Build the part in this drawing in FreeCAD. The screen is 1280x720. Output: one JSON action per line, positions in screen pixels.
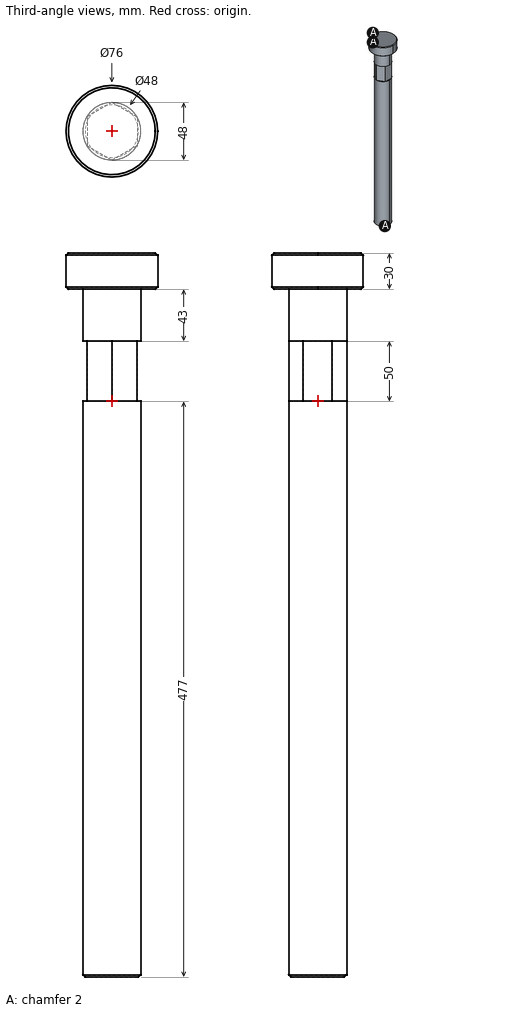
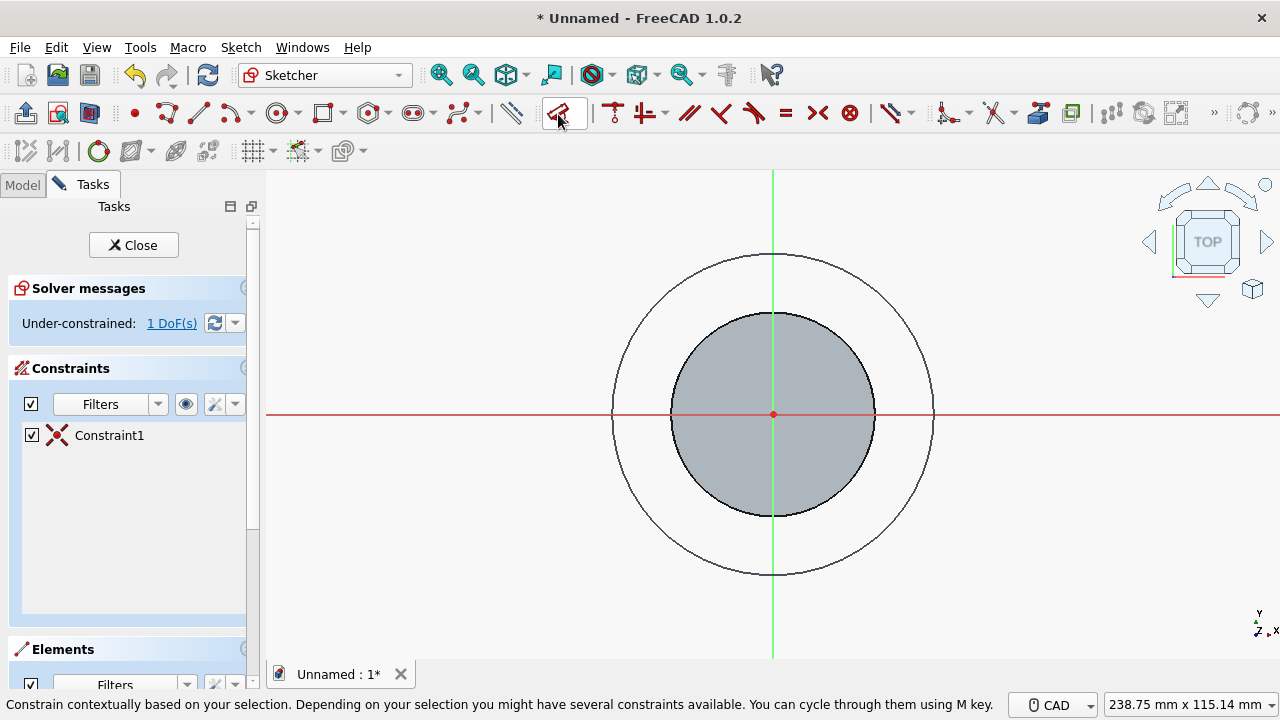
{"action": "left_click", "coordinate": [886, 300]}
{"action": "left_click", "coordinate": [908, 277]}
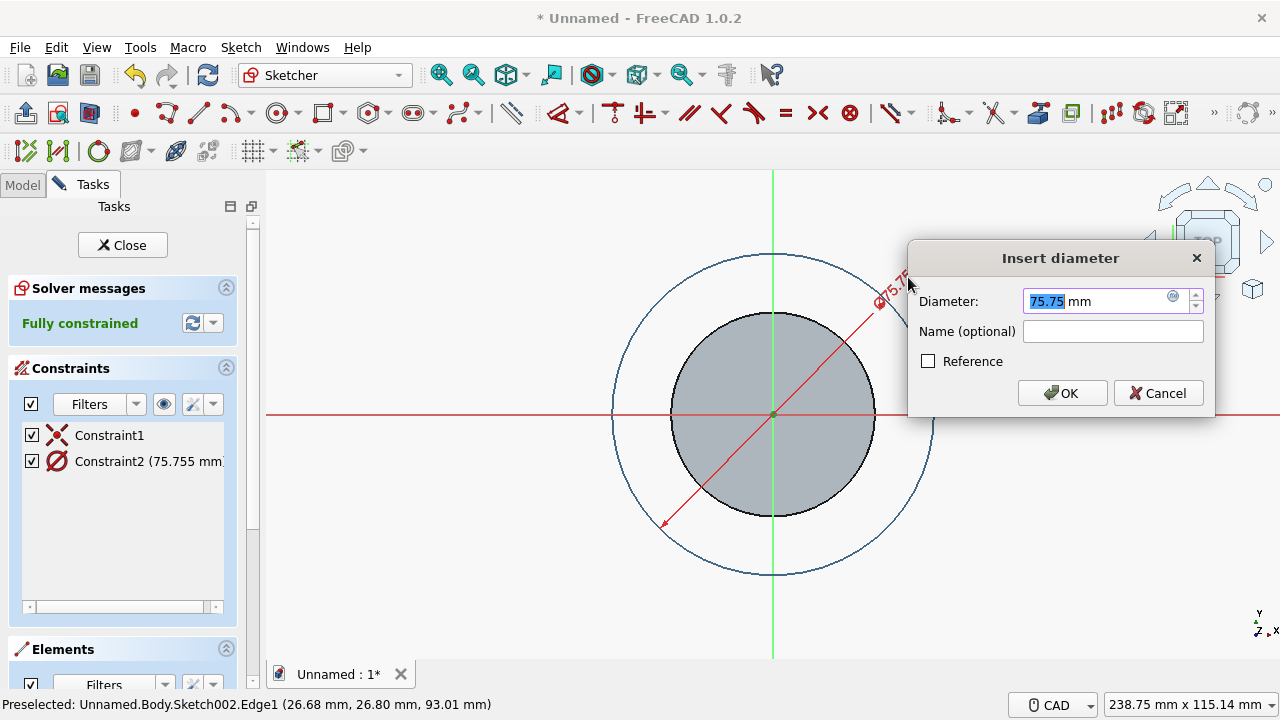
{"action": "type", "text": "76"}
{"action": "key", "text": "Return"}
{"action": "key", "text": "Escape"}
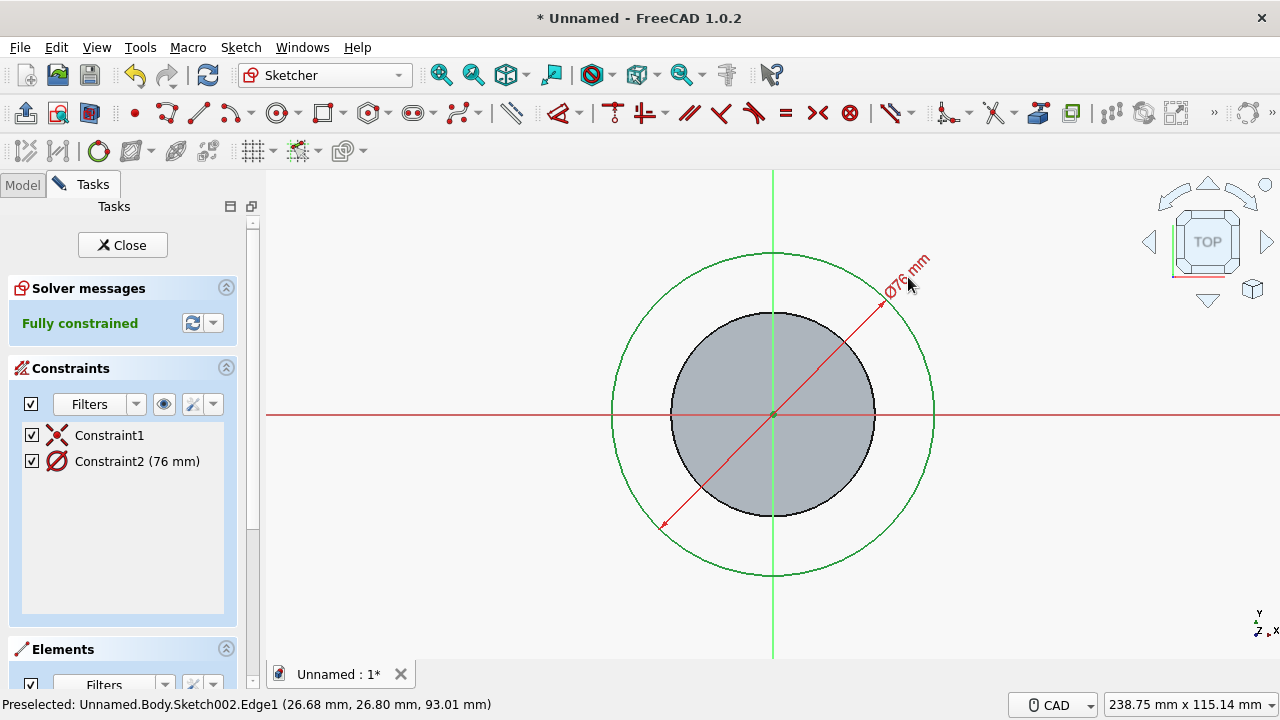
{"action": "left_click", "coordinate": [123, 245]}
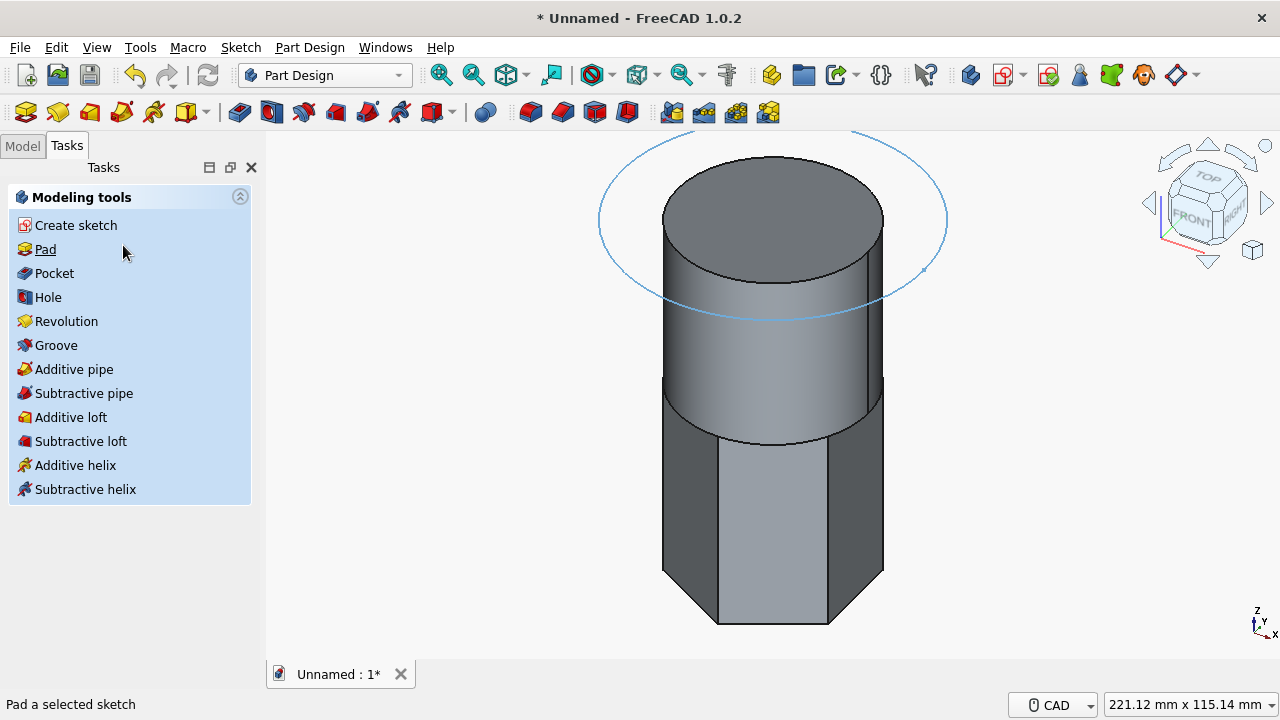
{"action": "left_click", "coordinate": [26, 112]}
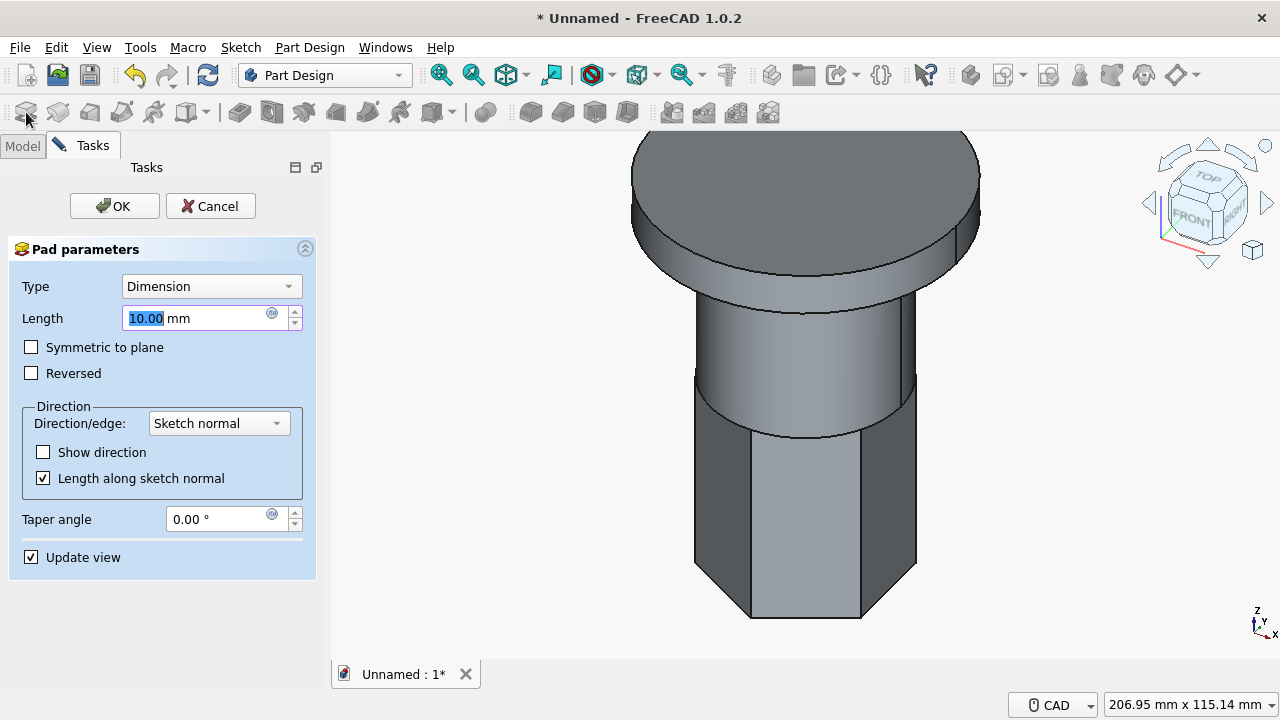
{"action": "type", "text": "30"}
{"action": "key", "text": "Tab"}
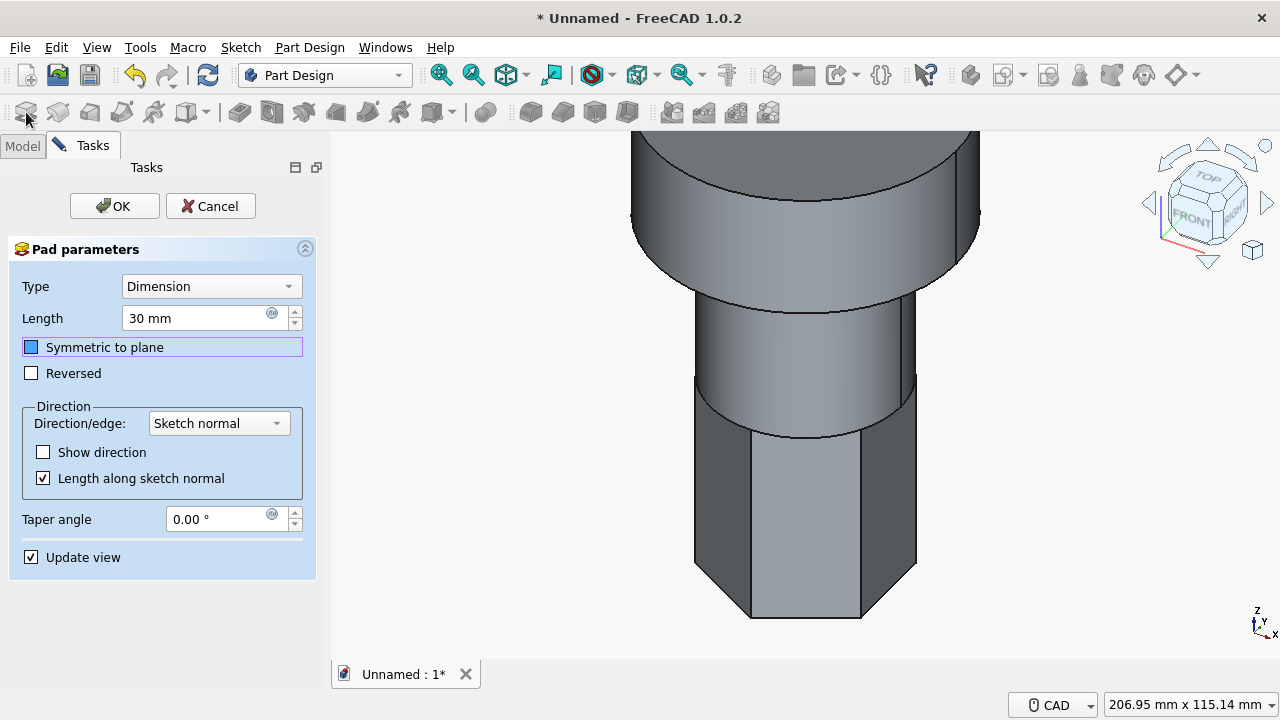
{"action": "left_click", "coordinate": [115, 206]}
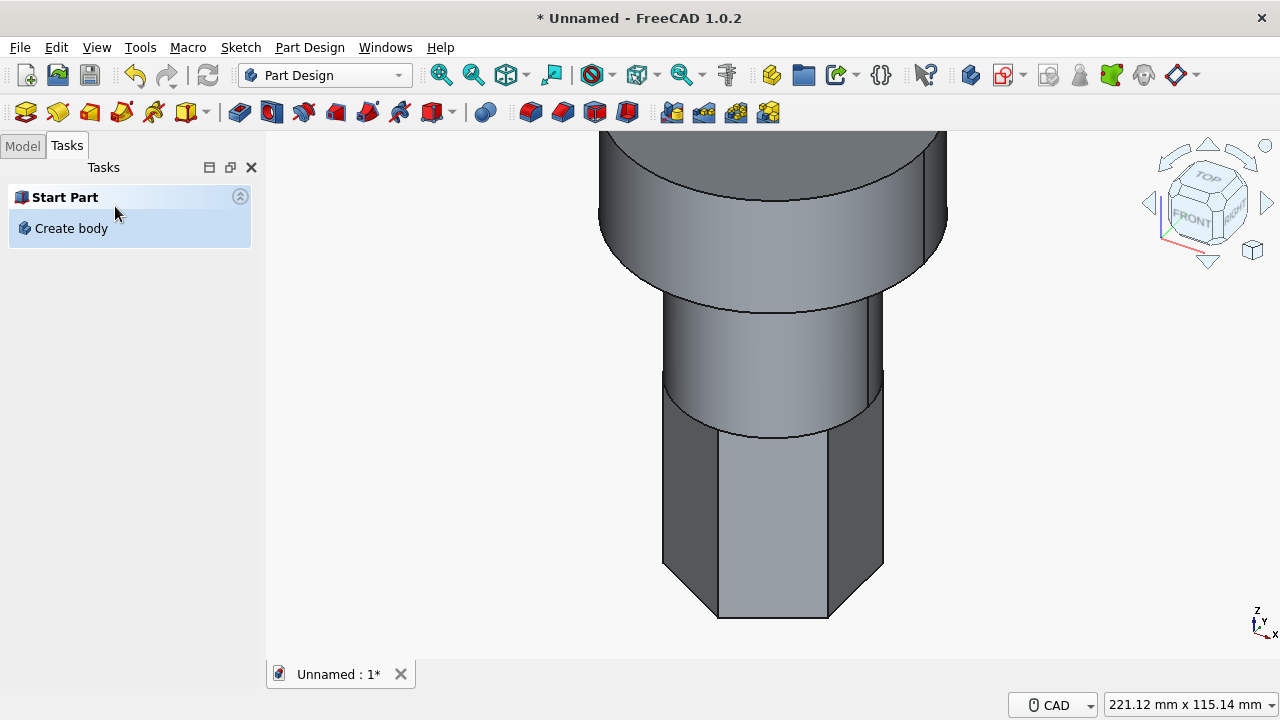
{"action": "key", "text": "v f"}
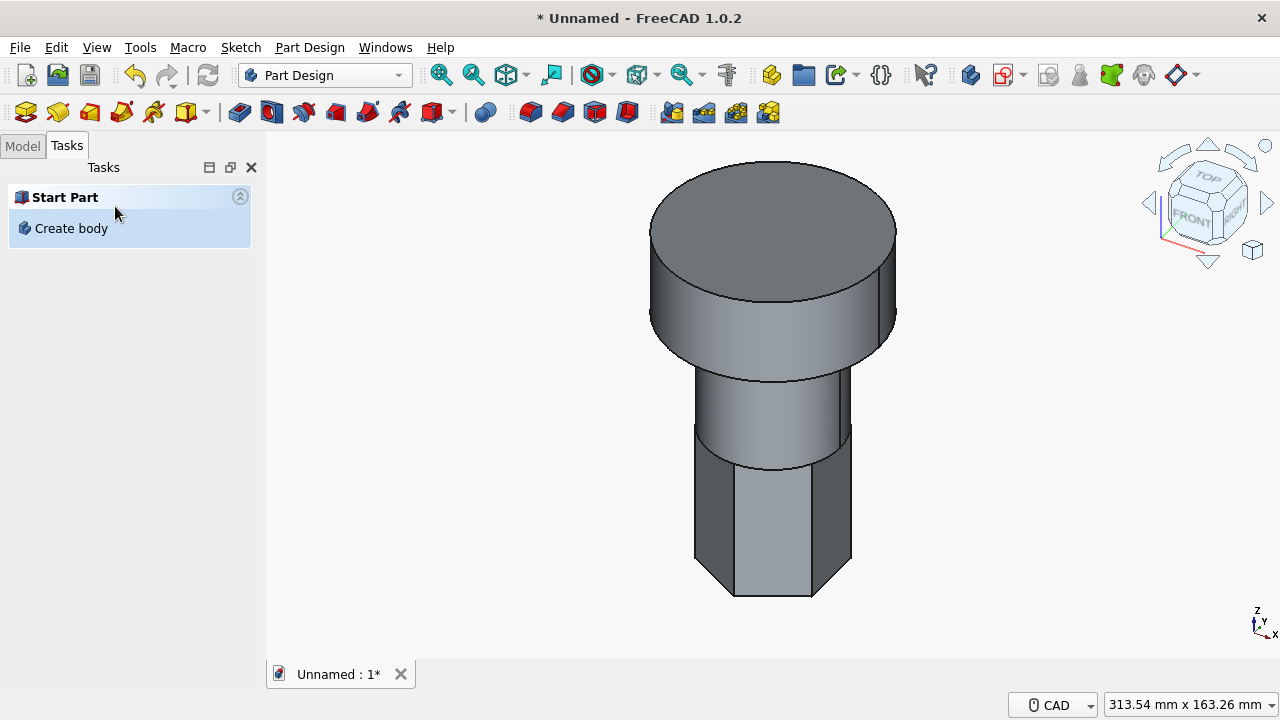
{"action": "left_click", "coordinate": [23, 145]}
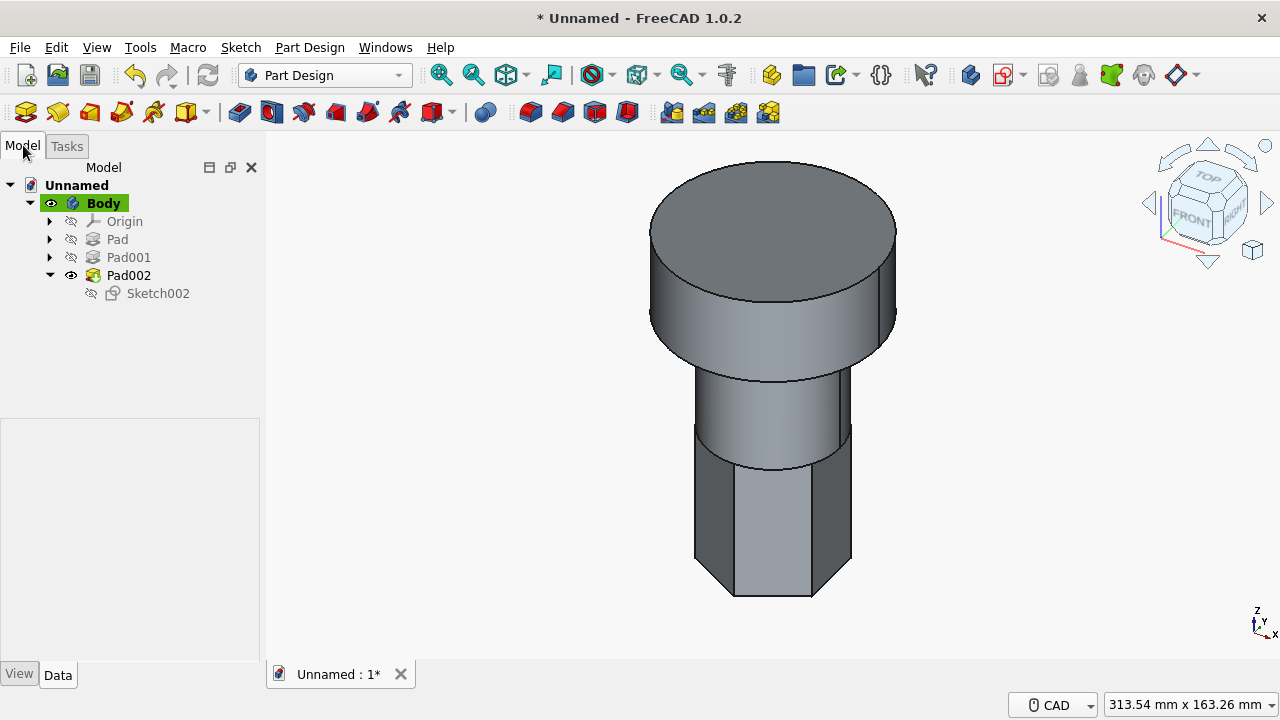
{"action": "left_click", "coordinate": [50, 221]}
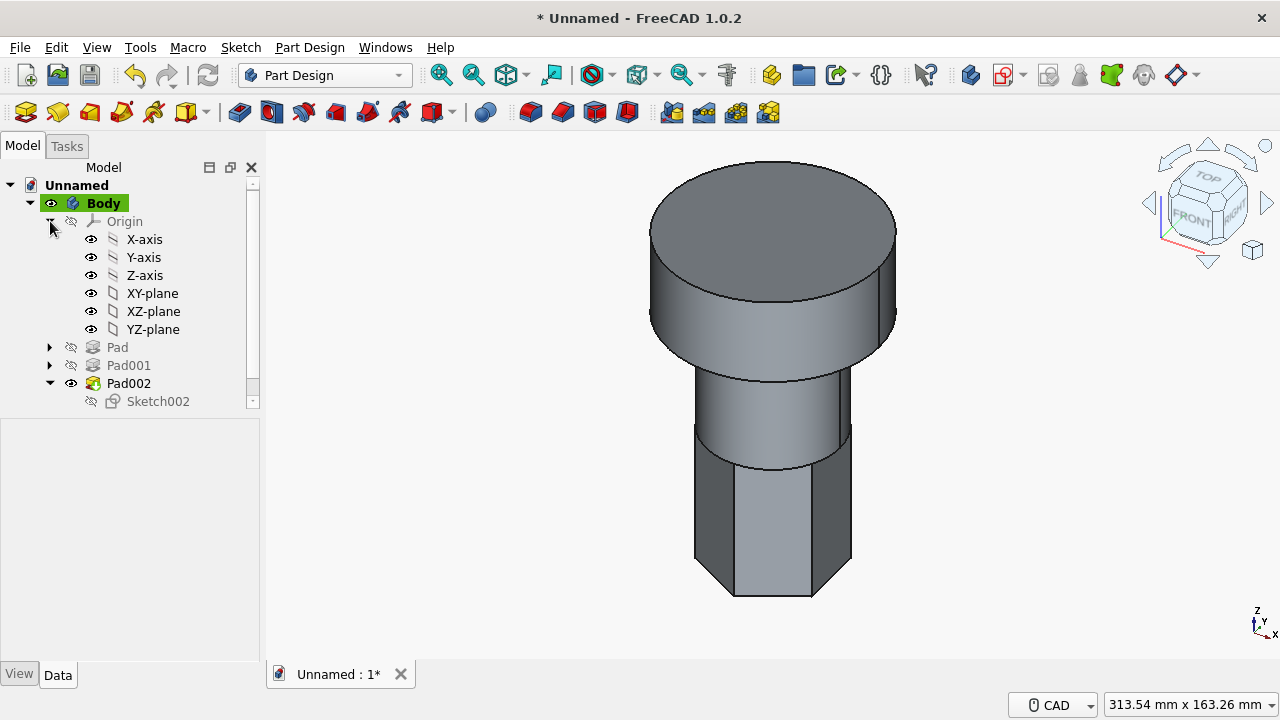
{"action": "left_click", "coordinate": [136, 293]}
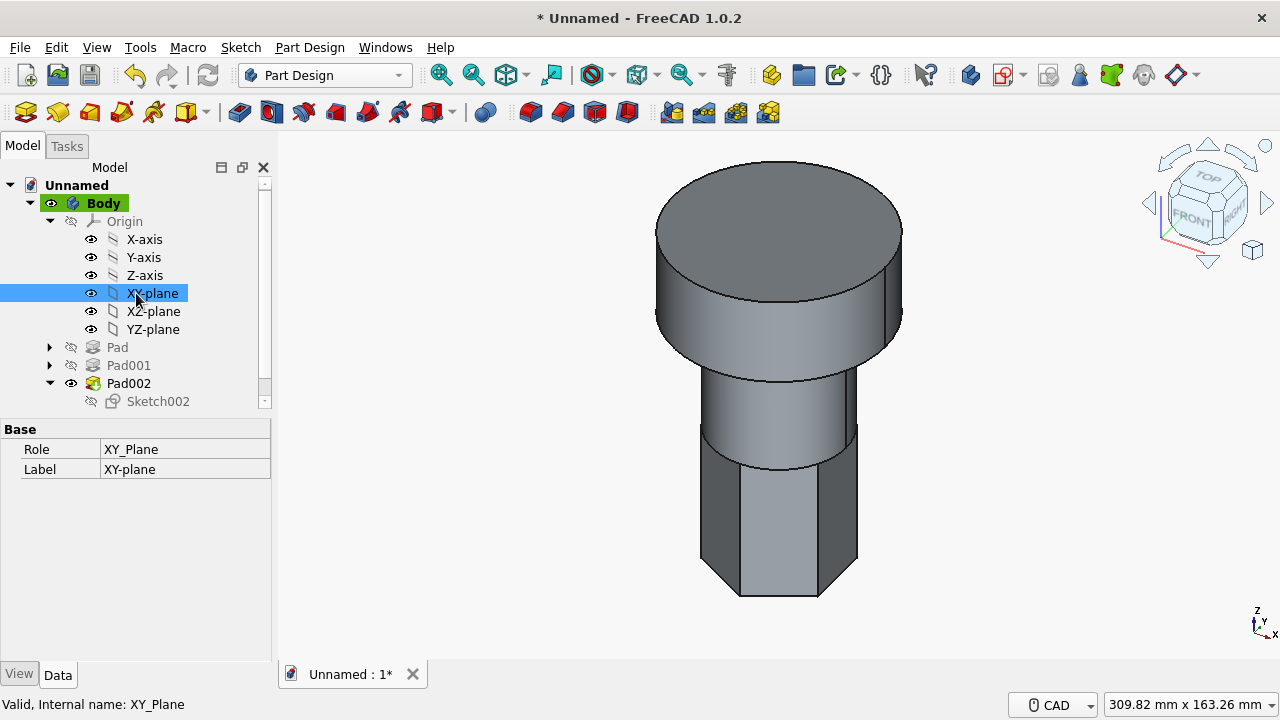
{"action": "left_click", "coordinate": [1176, 76]}